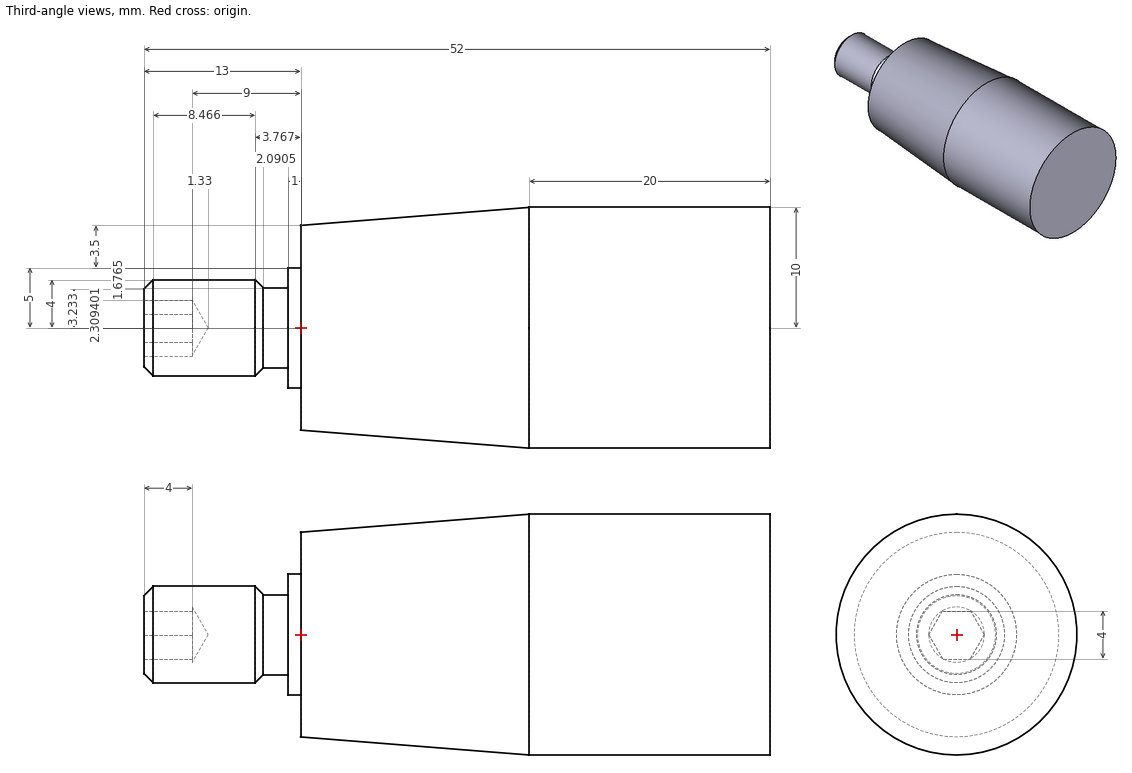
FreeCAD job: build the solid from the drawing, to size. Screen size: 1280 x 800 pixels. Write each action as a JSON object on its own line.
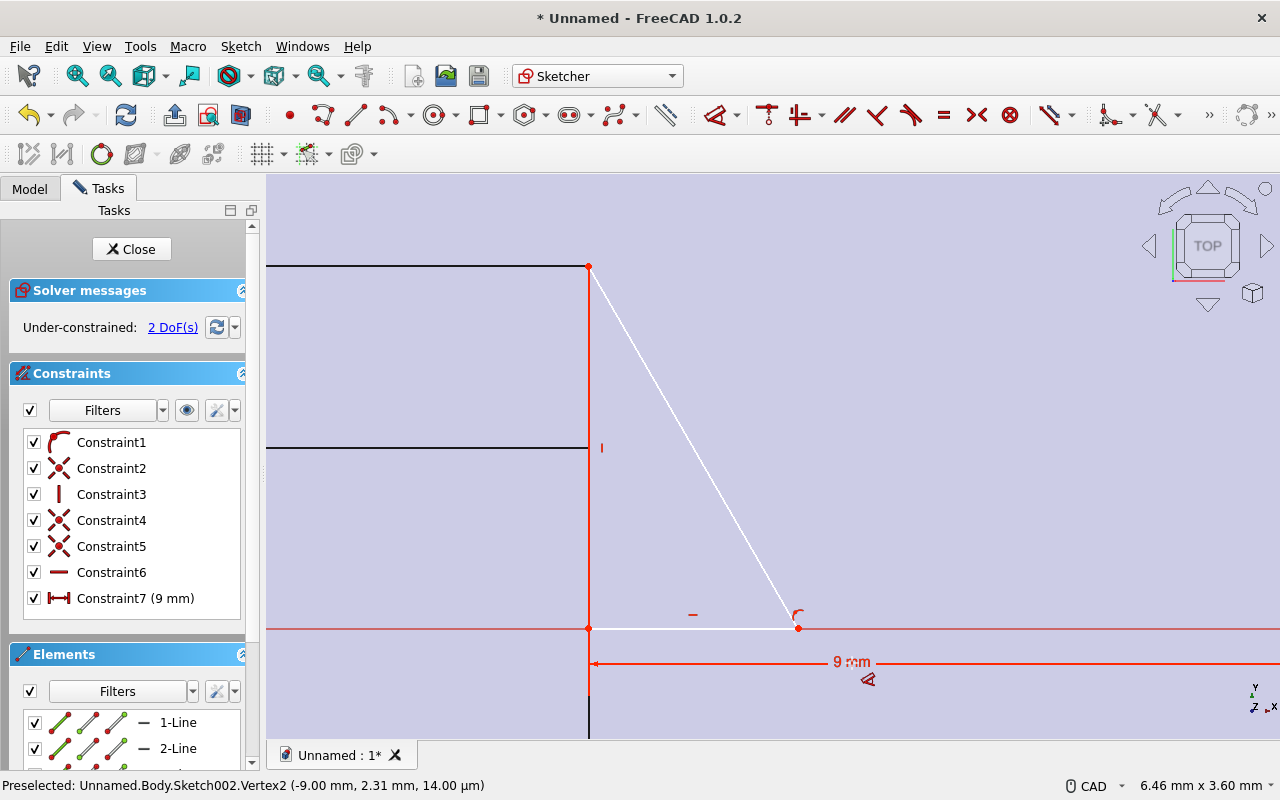
{"action": "left_click", "coordinate": [652, 629]}
{"action": "left_click", "coordinate": [693, 663]}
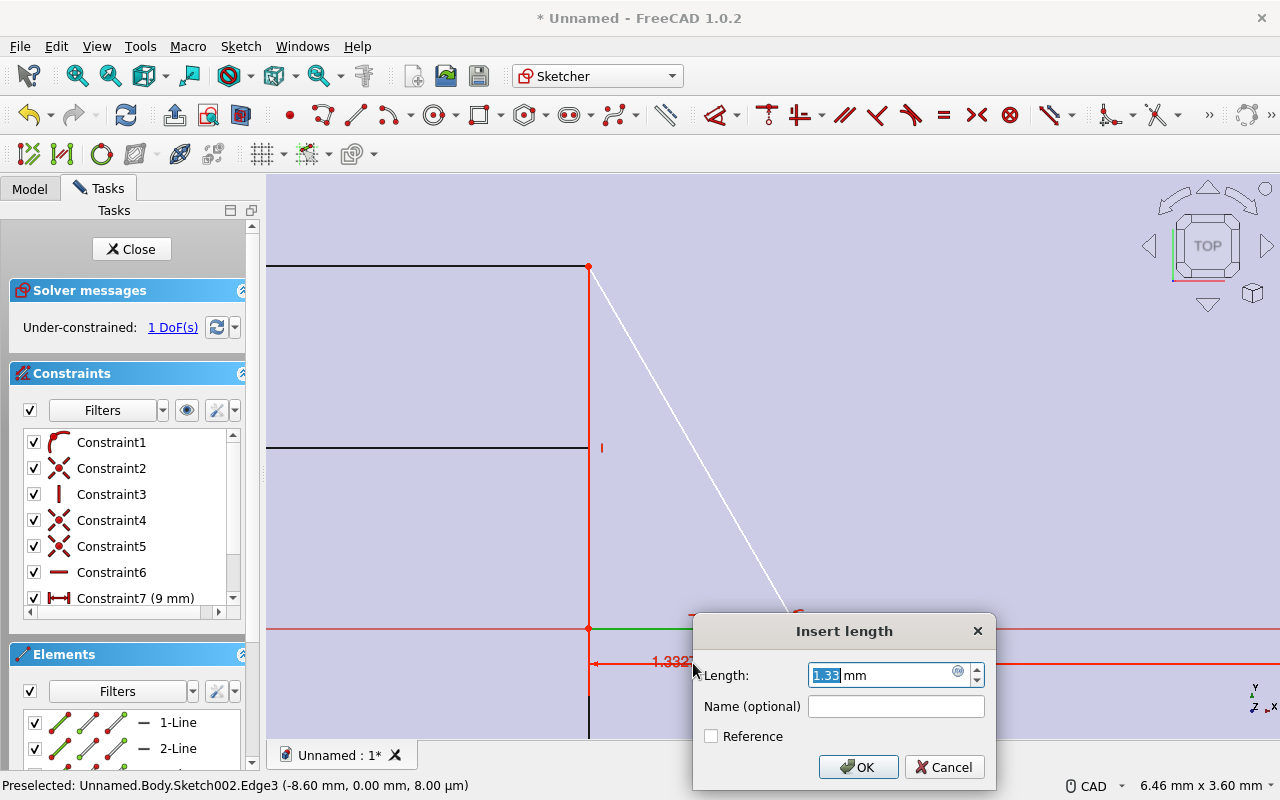
{"action": "type", "text": "1.33"}
{"action": "key", "text": "Return"}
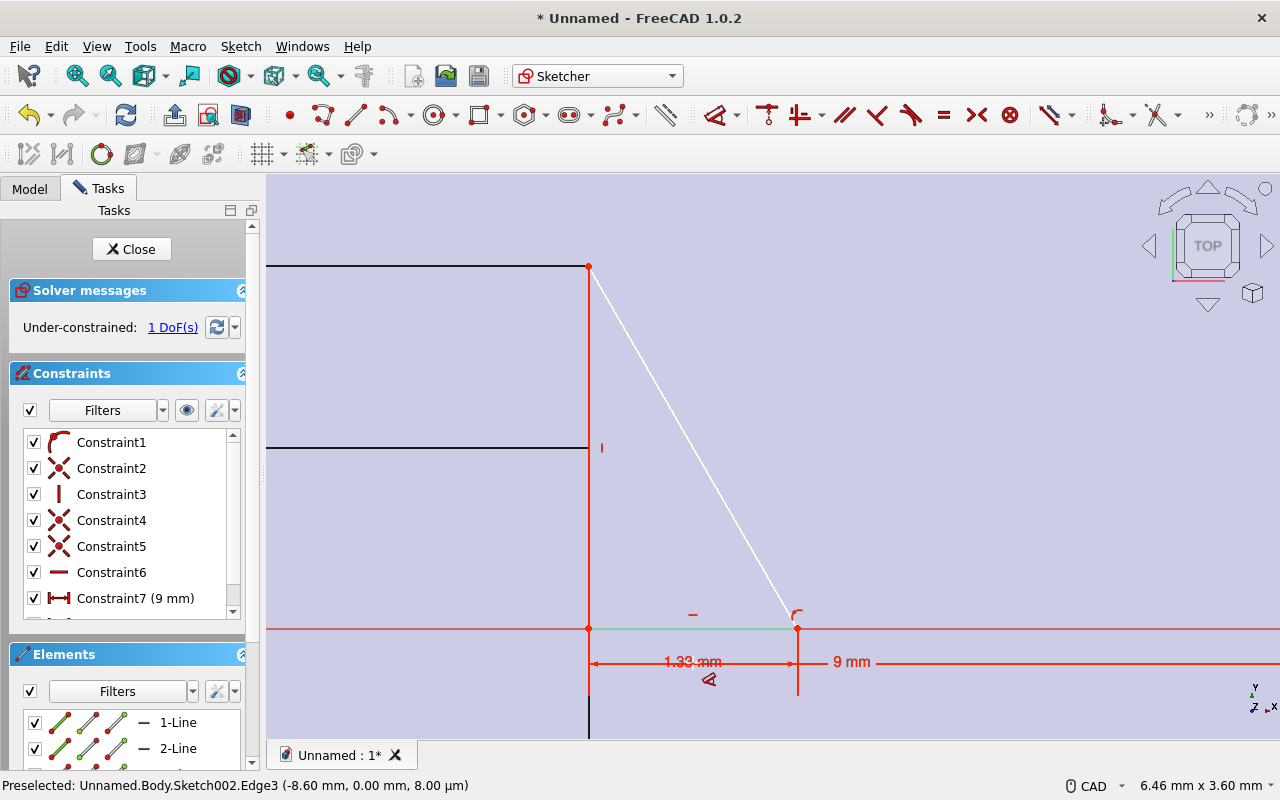
{"action": "left_click", "coordinate": [589, 376]}
{"action": "left_click", "coordinate": [555, 448]}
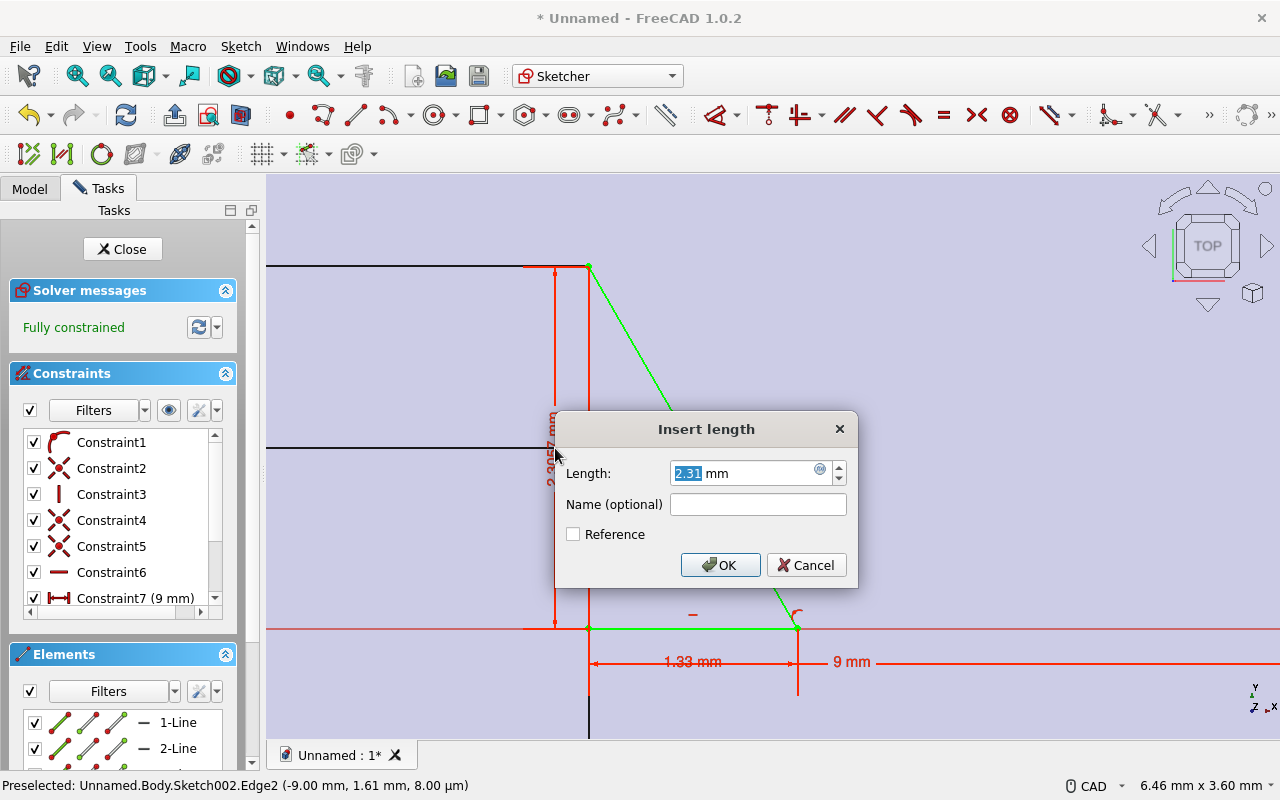
{"action": "type", "text": "2.309401"}
{"action": "key", "text": "Return"}
{"action": "key", "text": "Escape"}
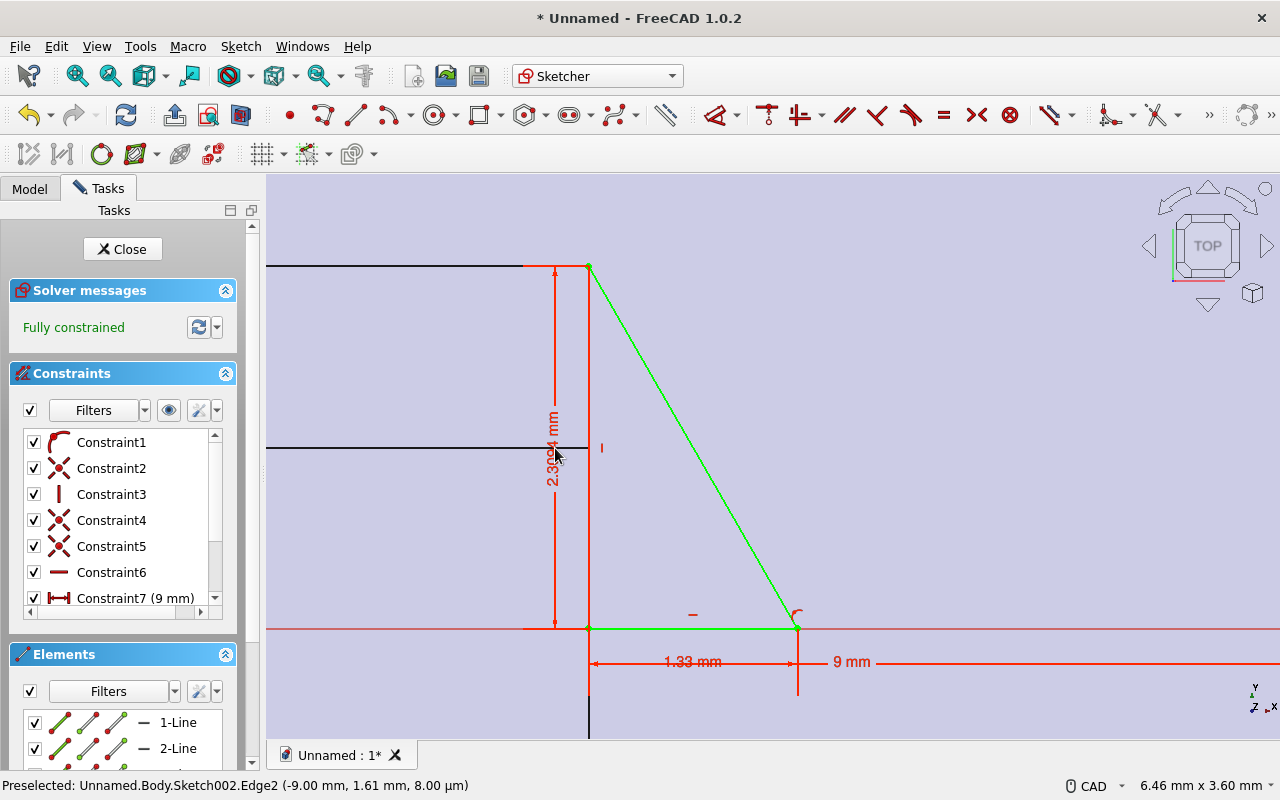
{"action": "left_click", "coordinate": [123, 249]}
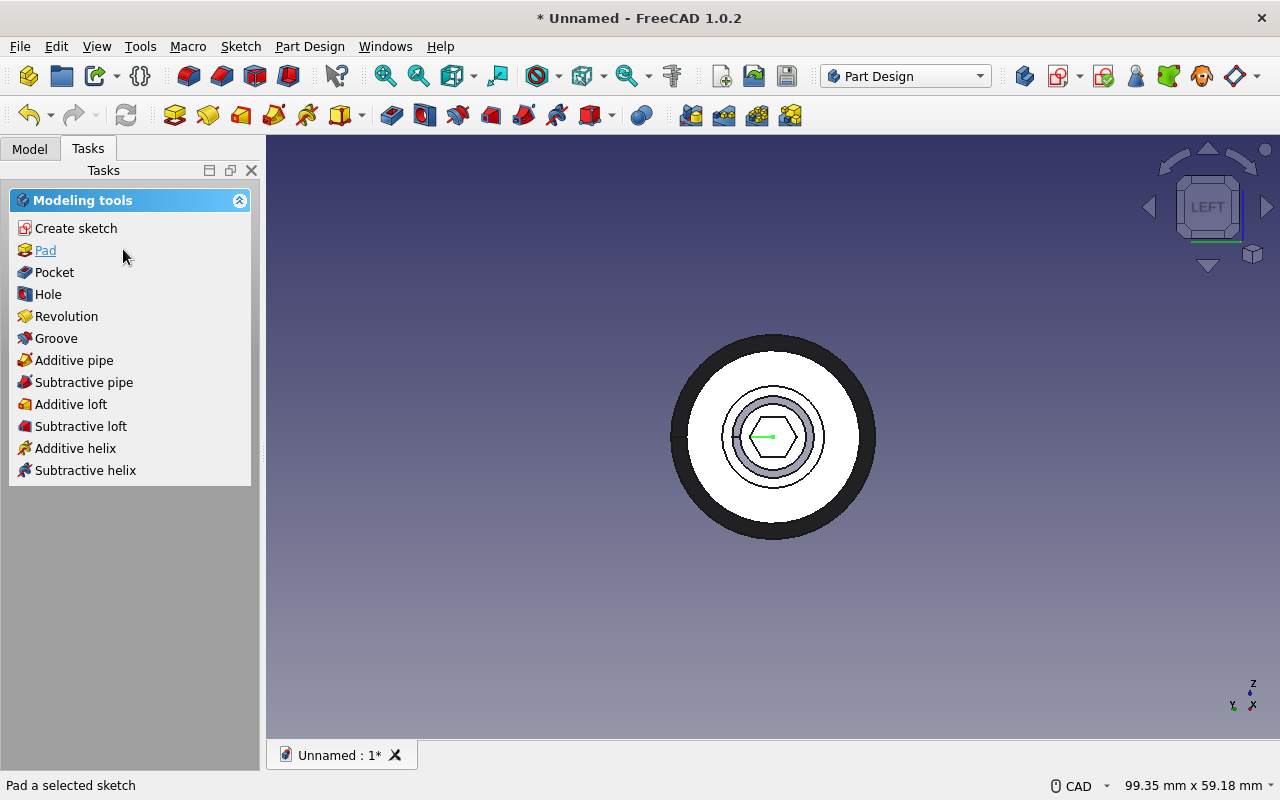
{"action": "left_click", "coordinate": [458, 116]}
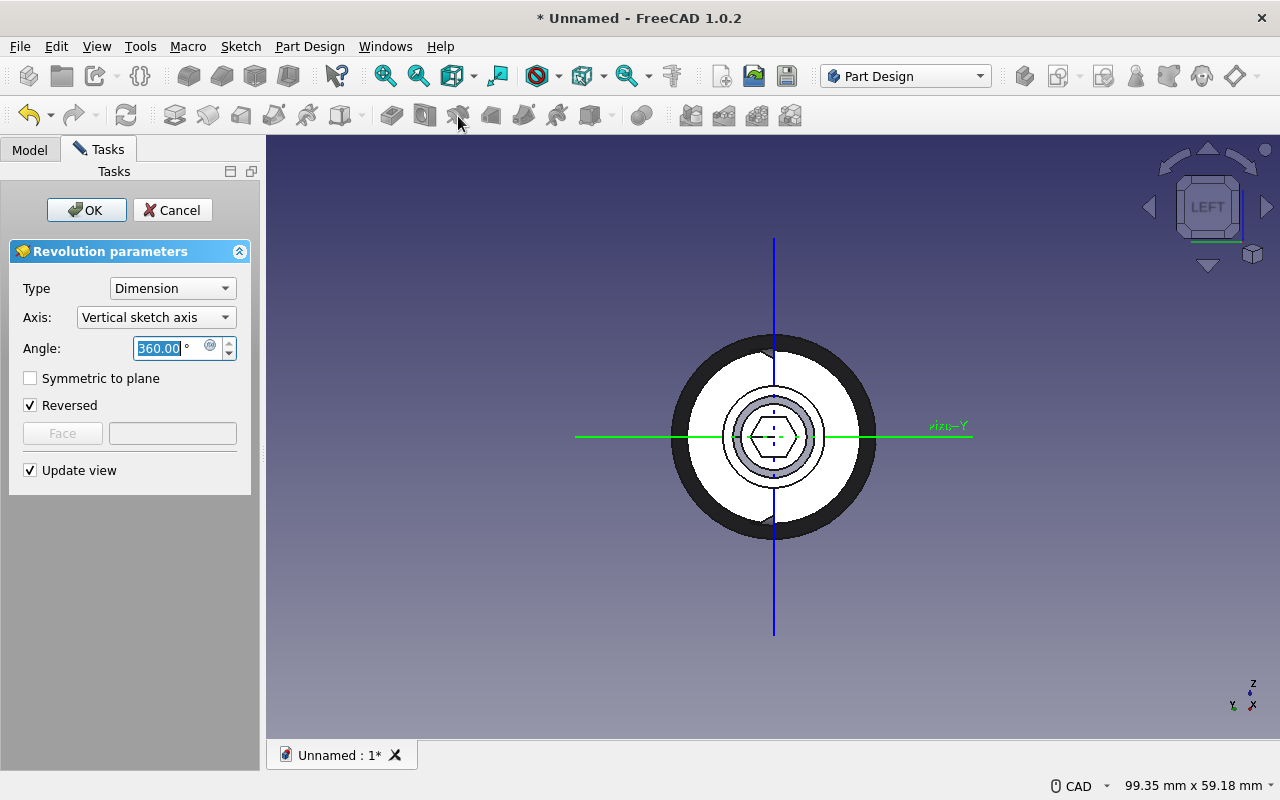
{"action": "left_click", "coordinate": [157, 318]}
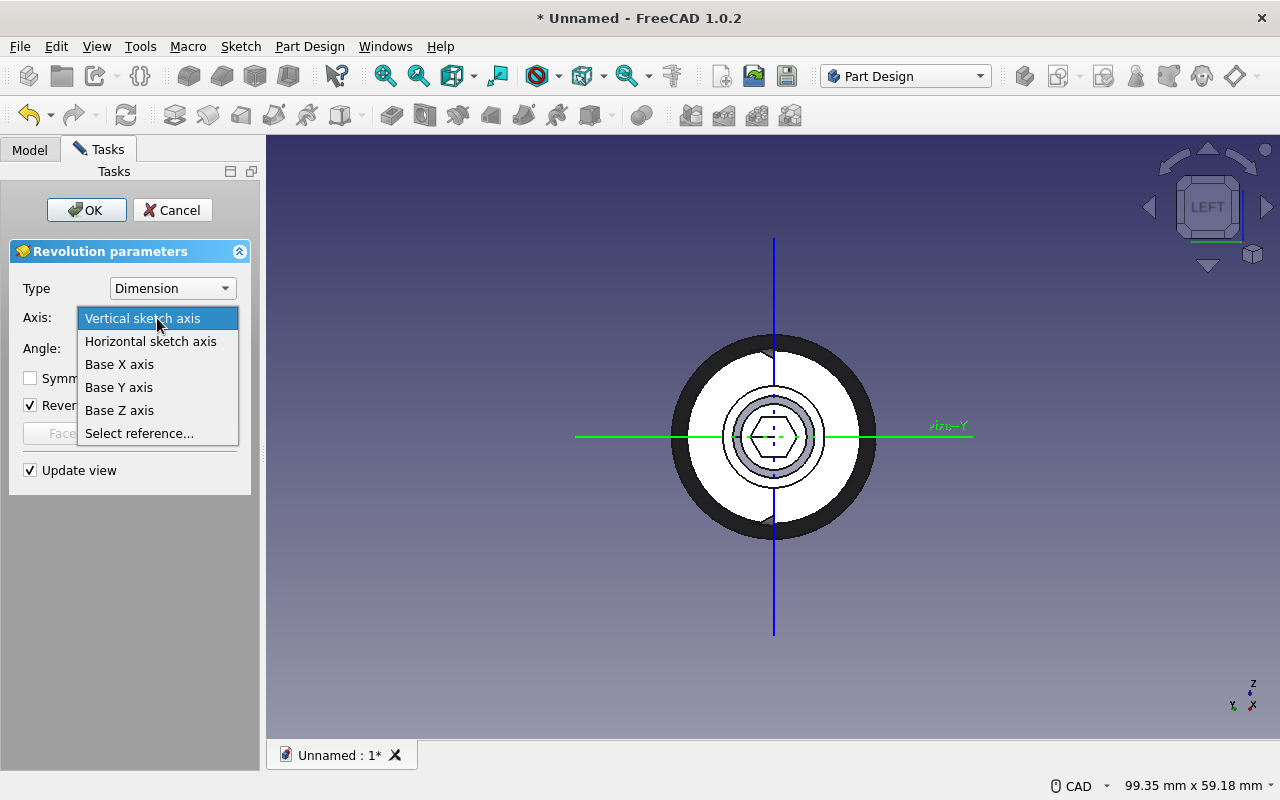
{"action": "left_click", "coordinate": [156, 342]}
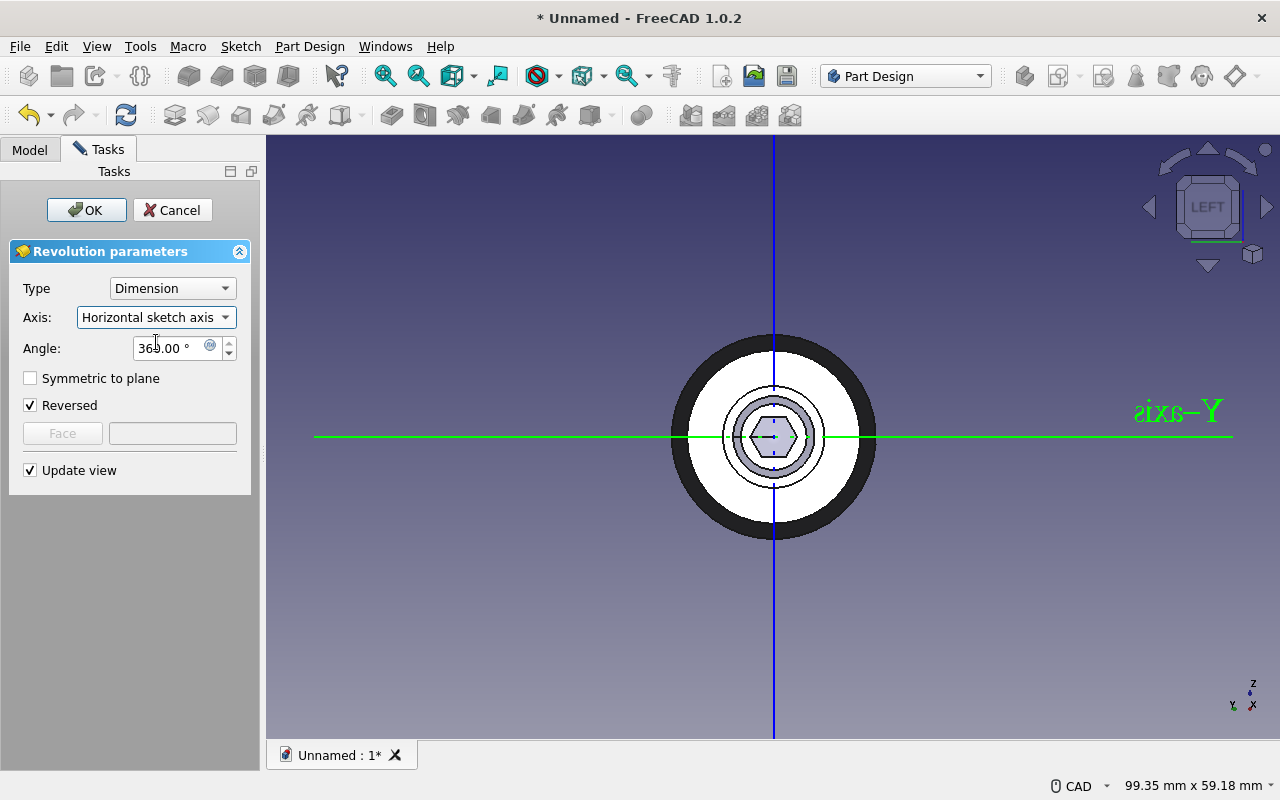
{"action": "left_click", "coordinate": [87, 210]}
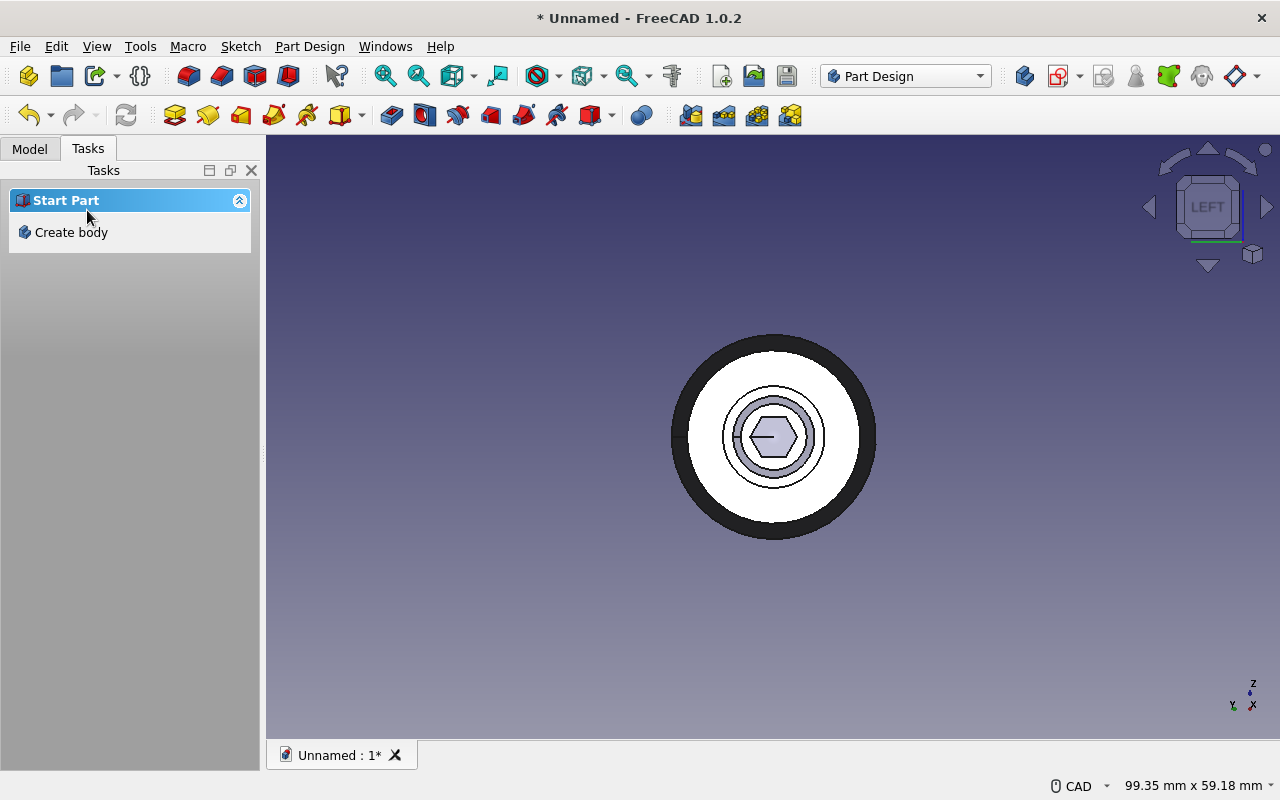
{"action": "key", "text": "0"}